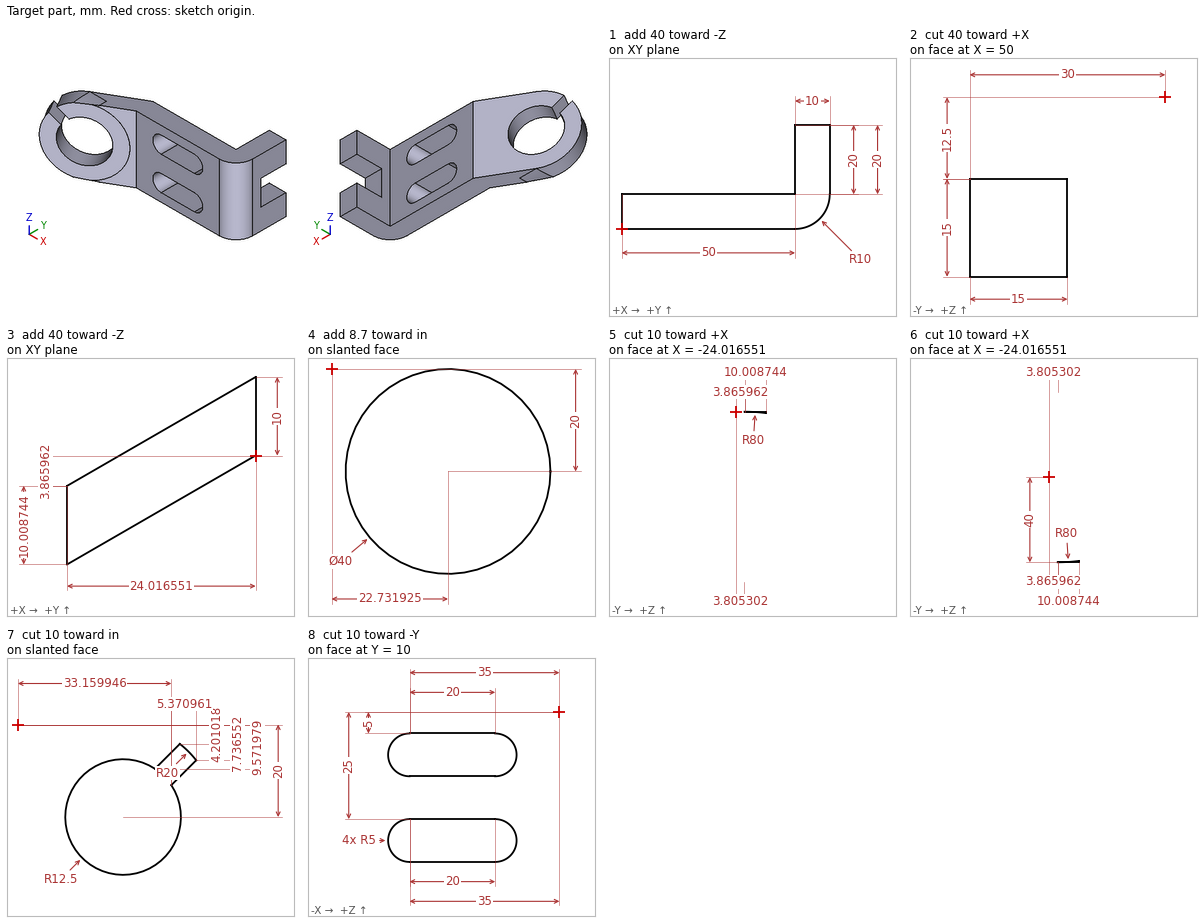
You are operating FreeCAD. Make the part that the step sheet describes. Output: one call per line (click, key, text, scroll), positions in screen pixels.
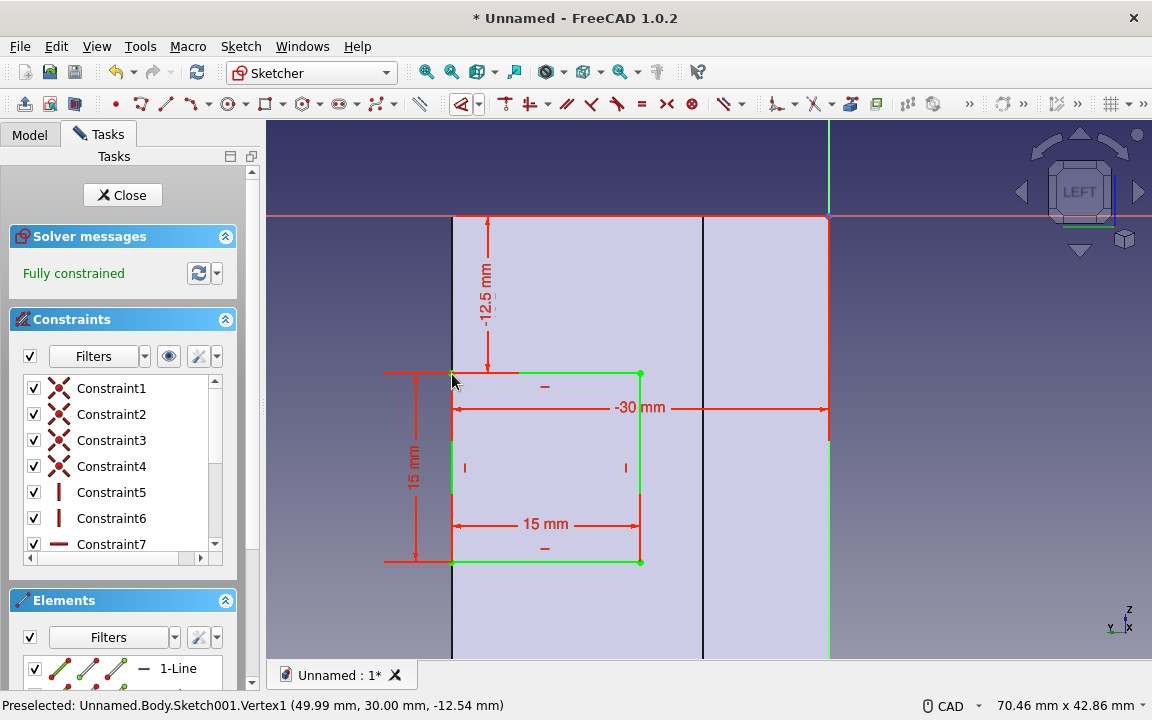
click(123, 195)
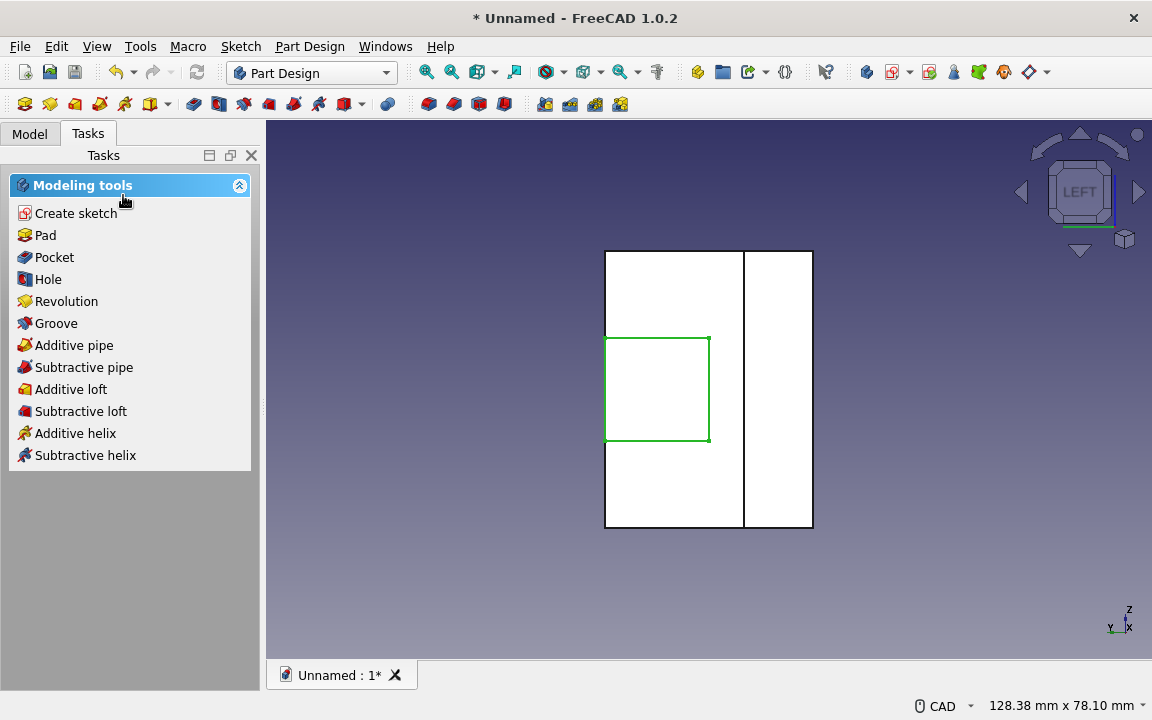
click(194, 104)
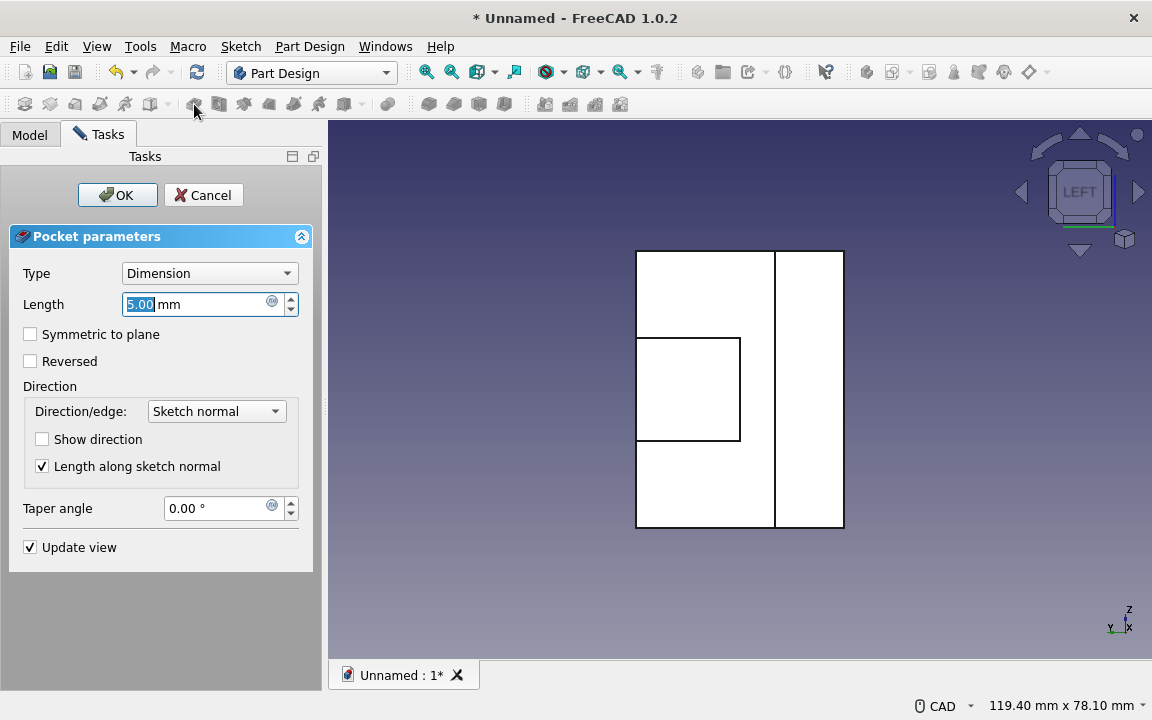
text(40)
key(Tab)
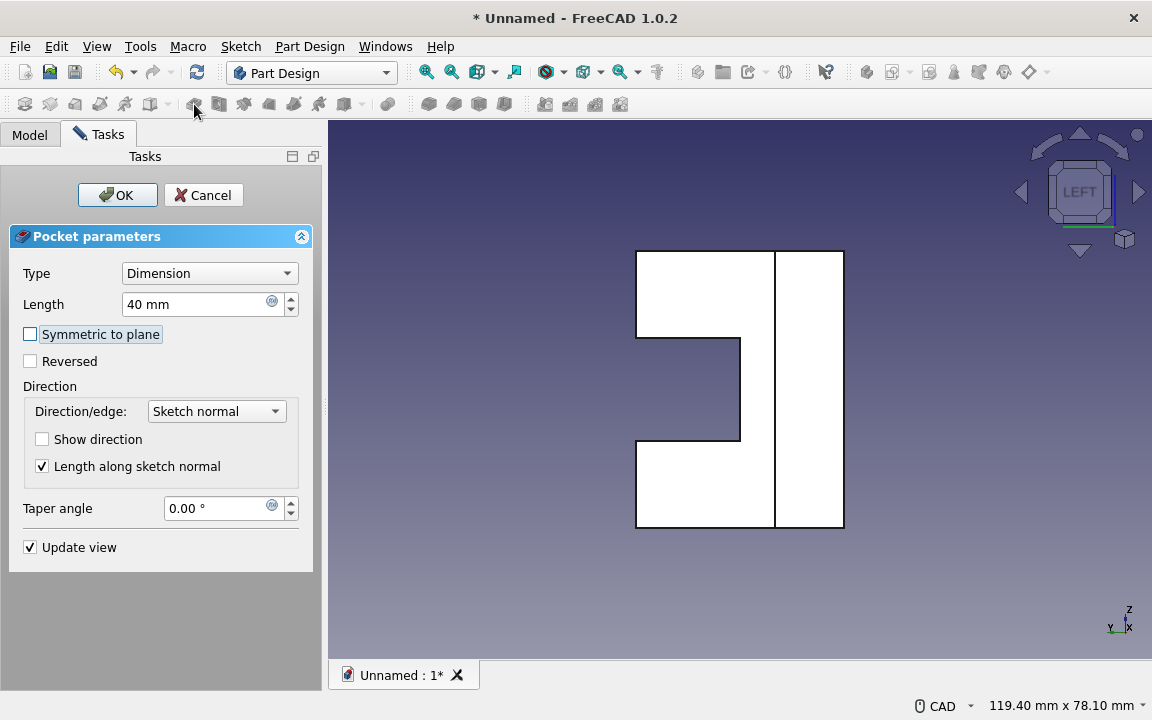
click(118, 195)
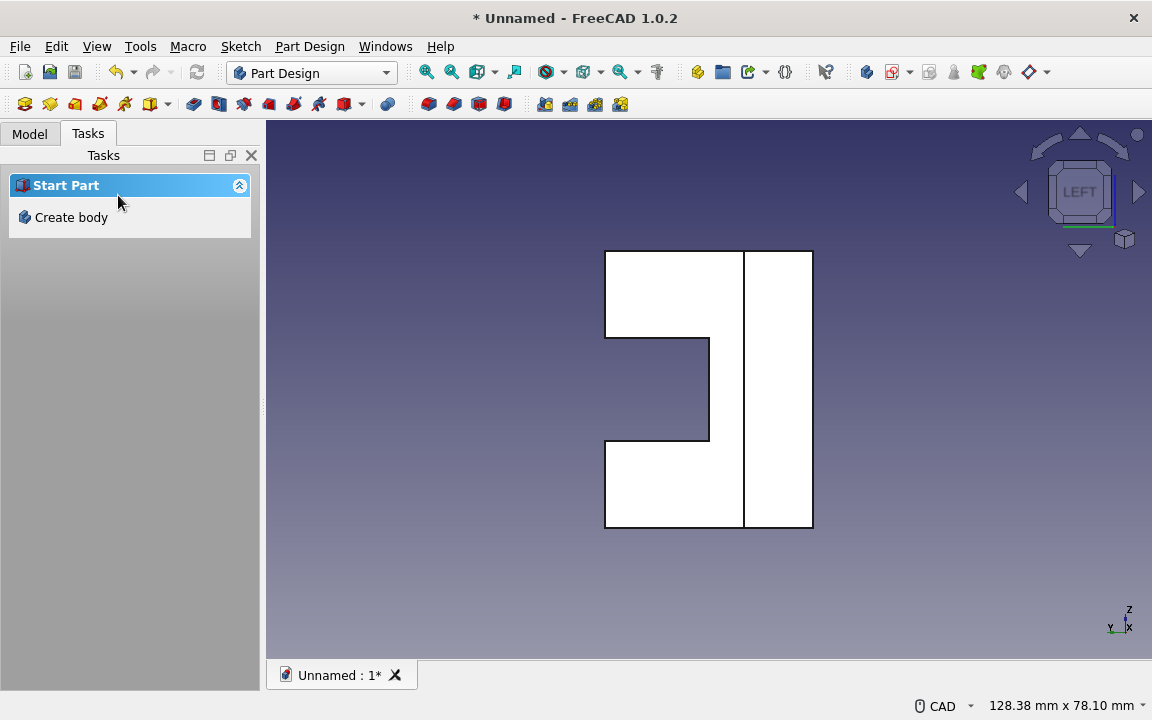
click(892, 72)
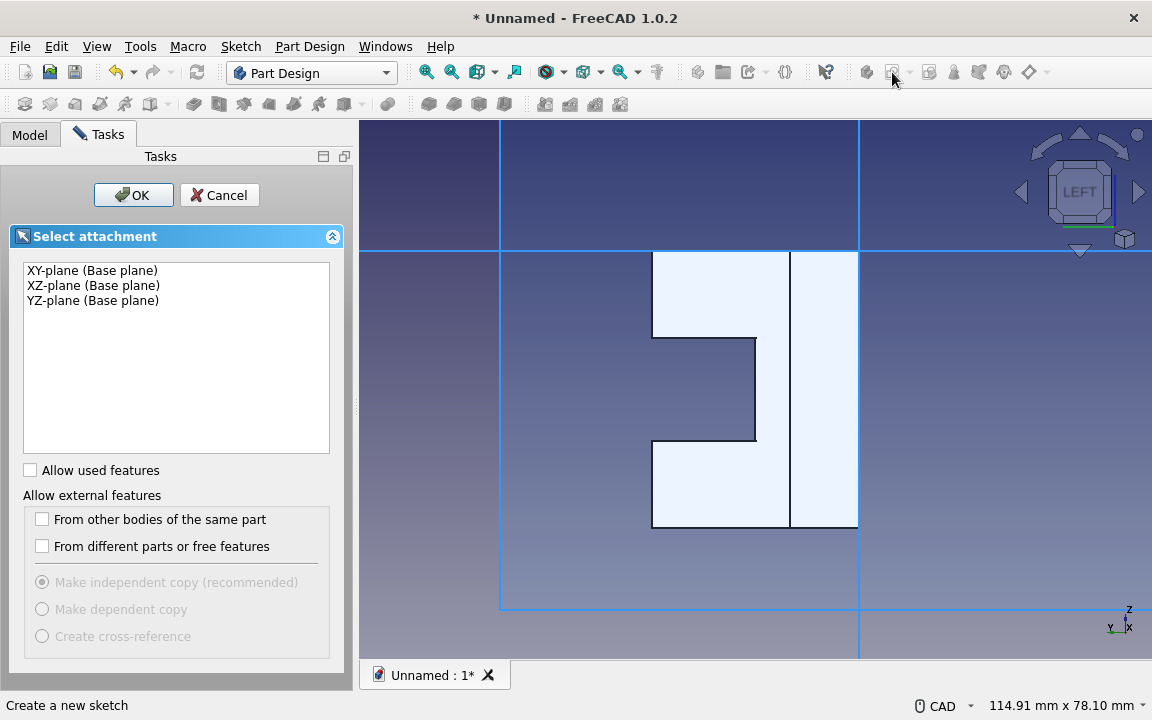
click(84, 270)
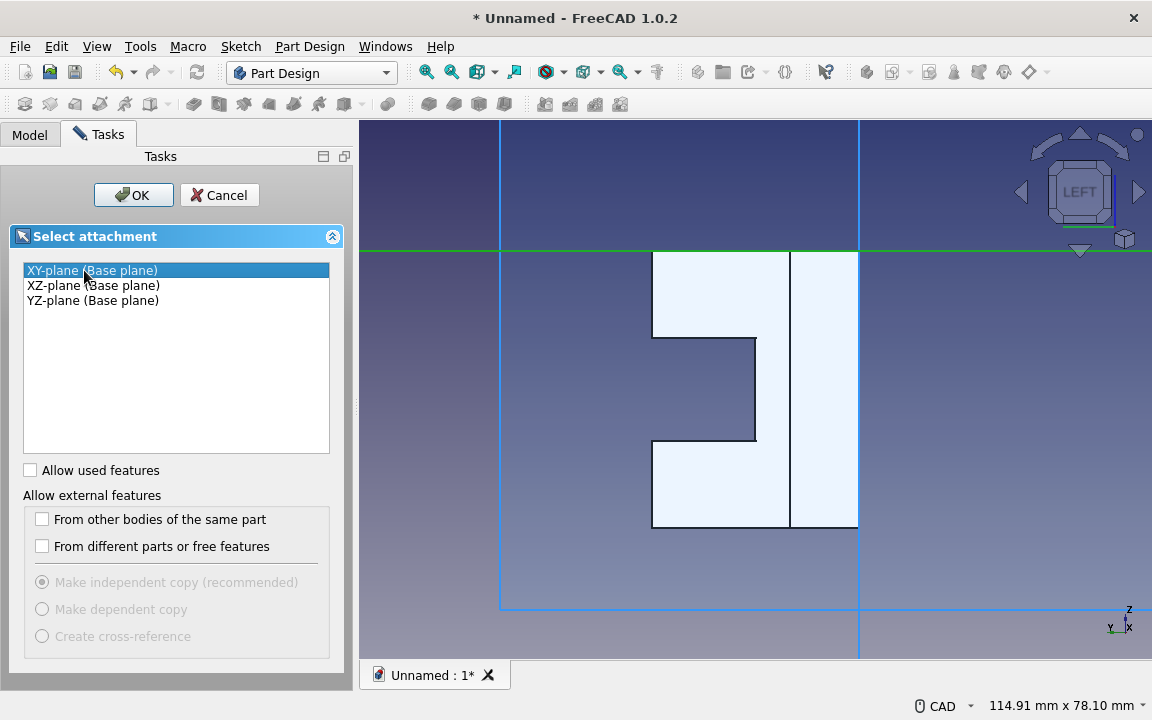
click(134, 195)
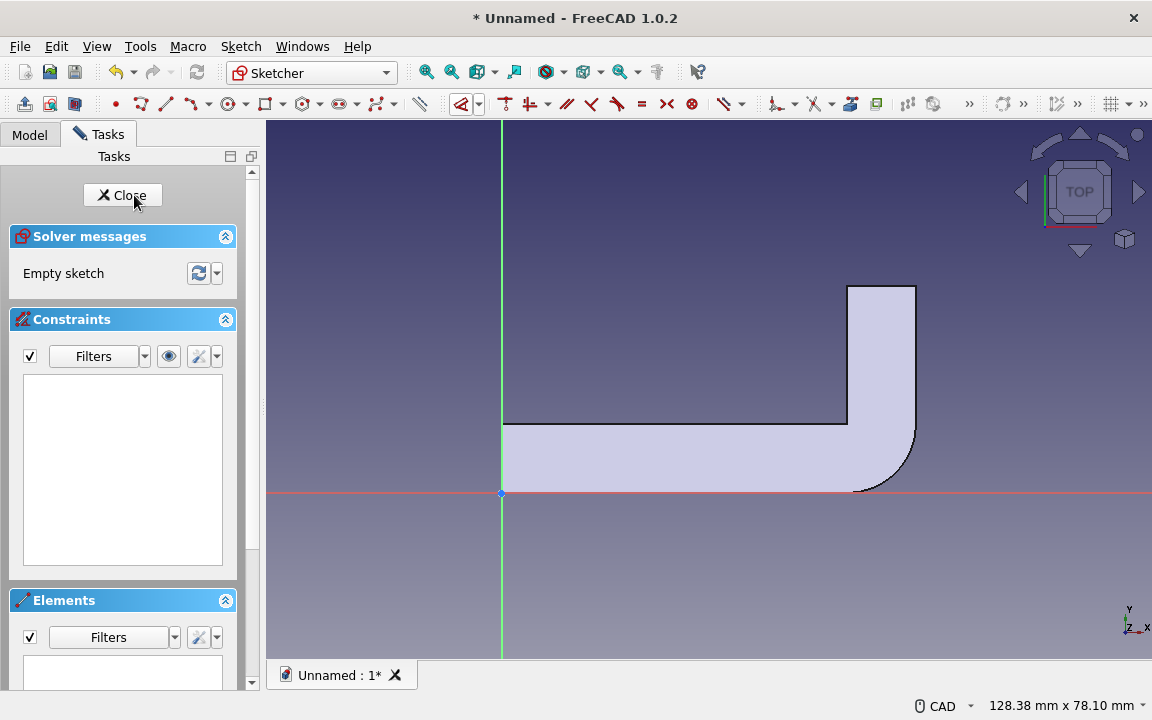
scroll(294, 602, up, 4)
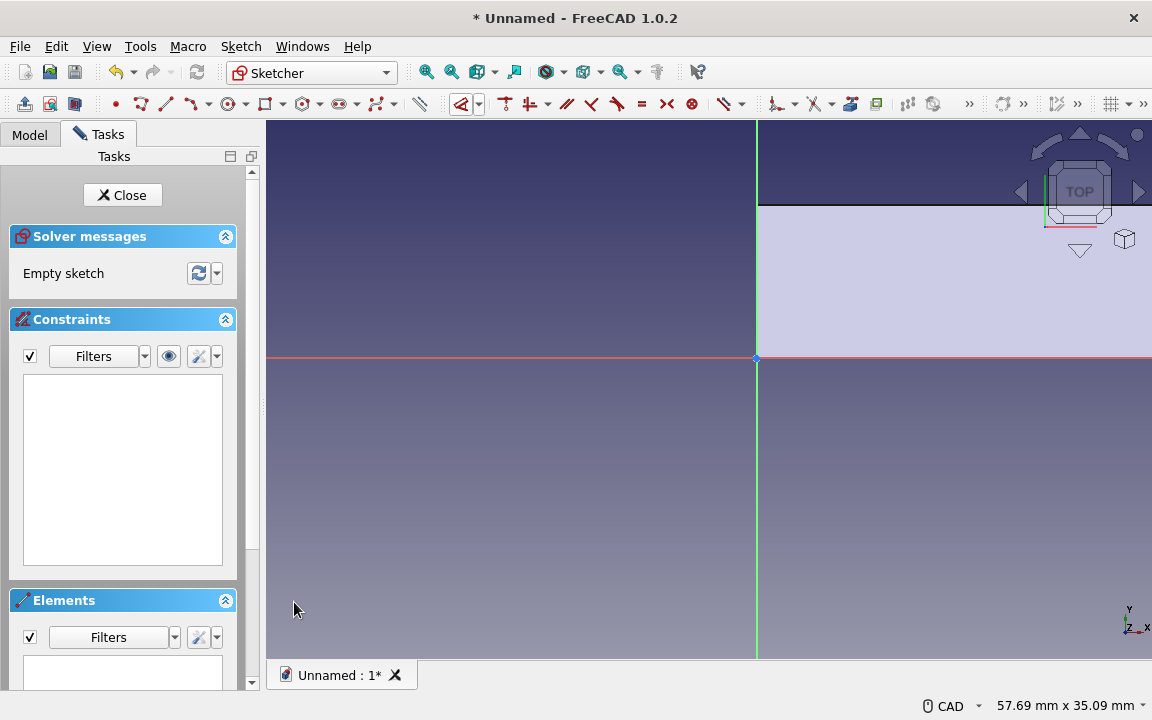
click(141, 104)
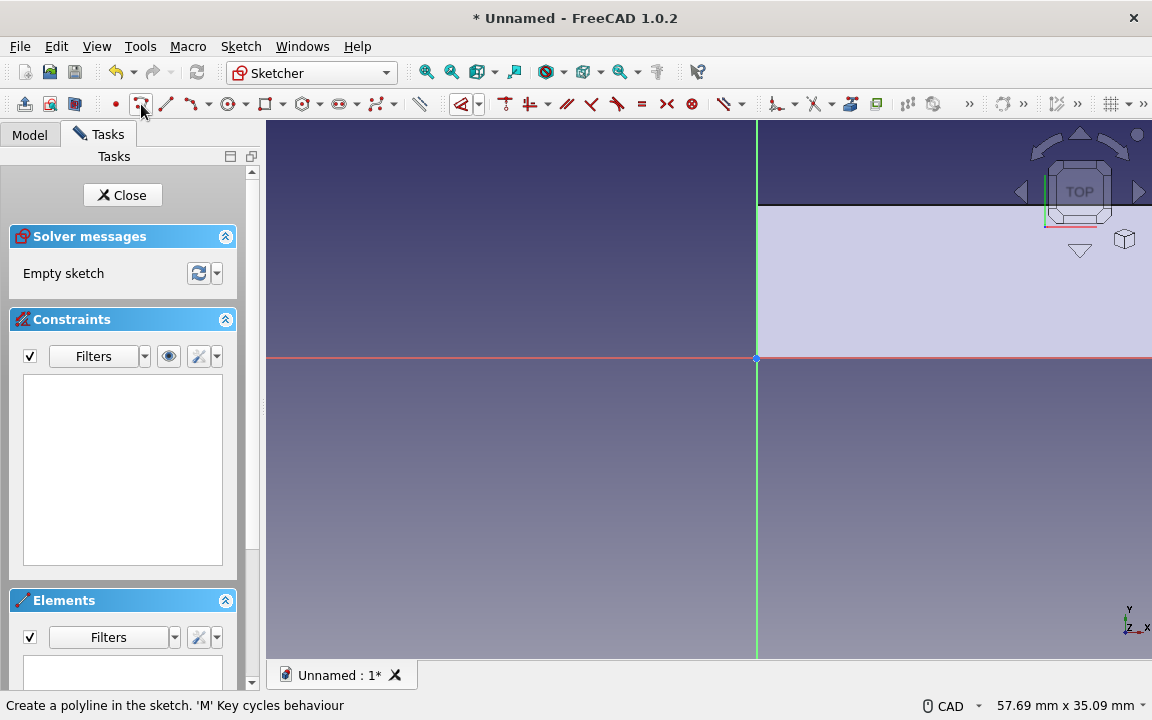
click(757, 358)
click(748, 205)
click(388, 418)
click(388, 571)
click(757, 358)
key(Escape)
key(Escape)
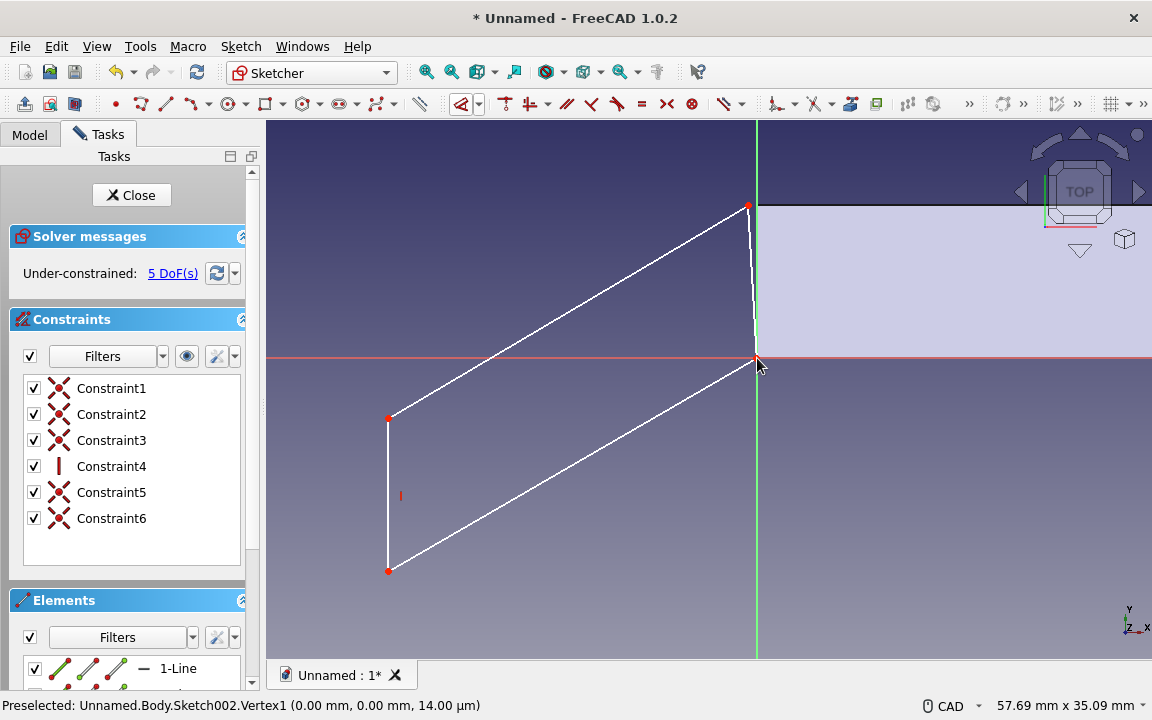
click(754, 313)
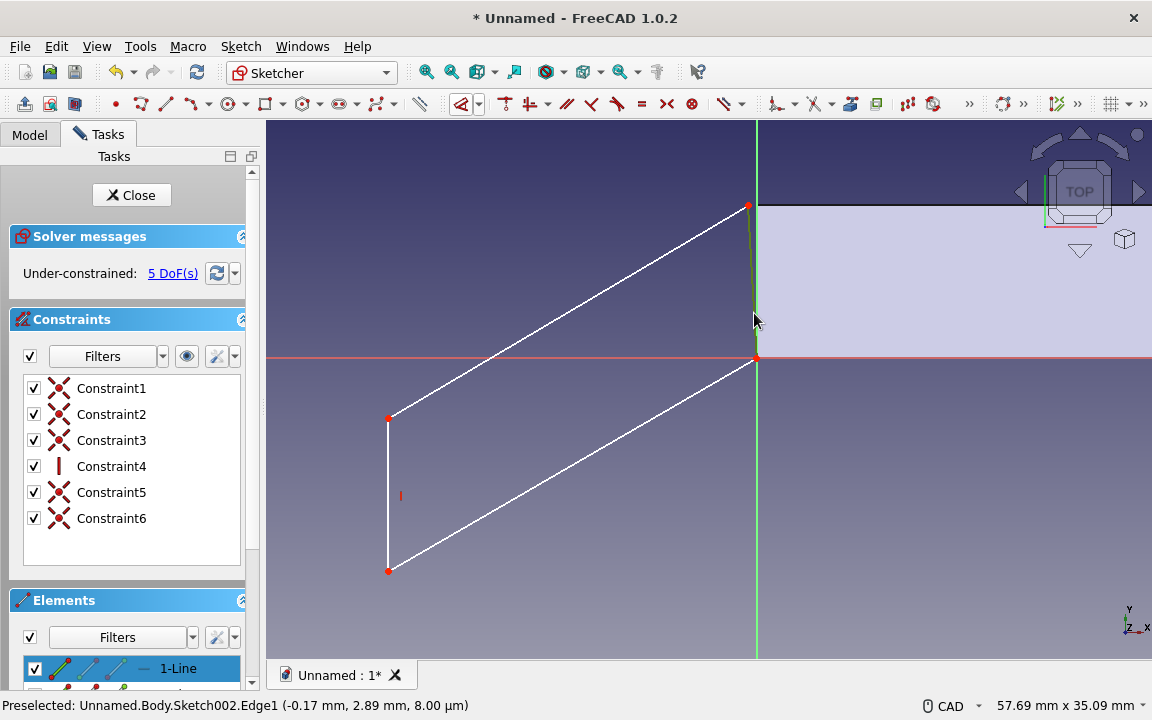
key(v)